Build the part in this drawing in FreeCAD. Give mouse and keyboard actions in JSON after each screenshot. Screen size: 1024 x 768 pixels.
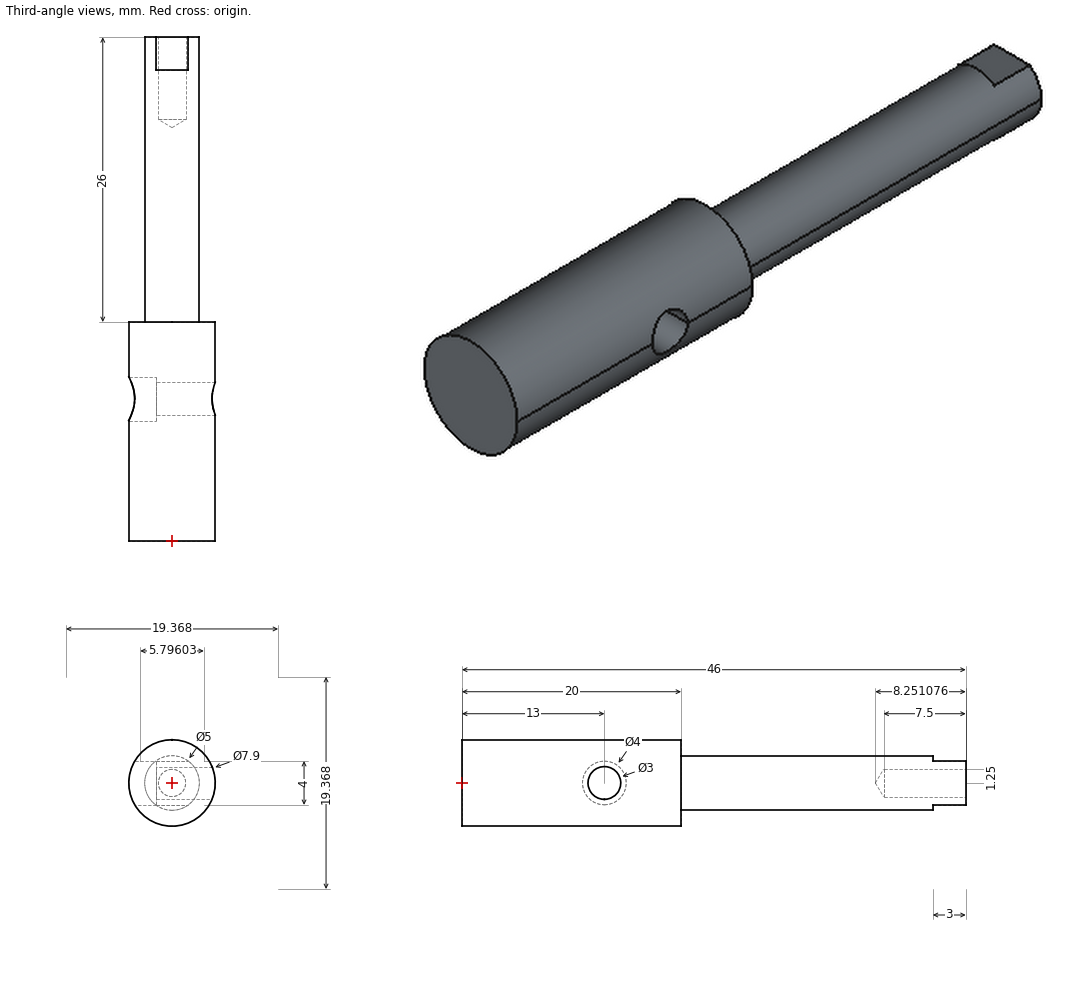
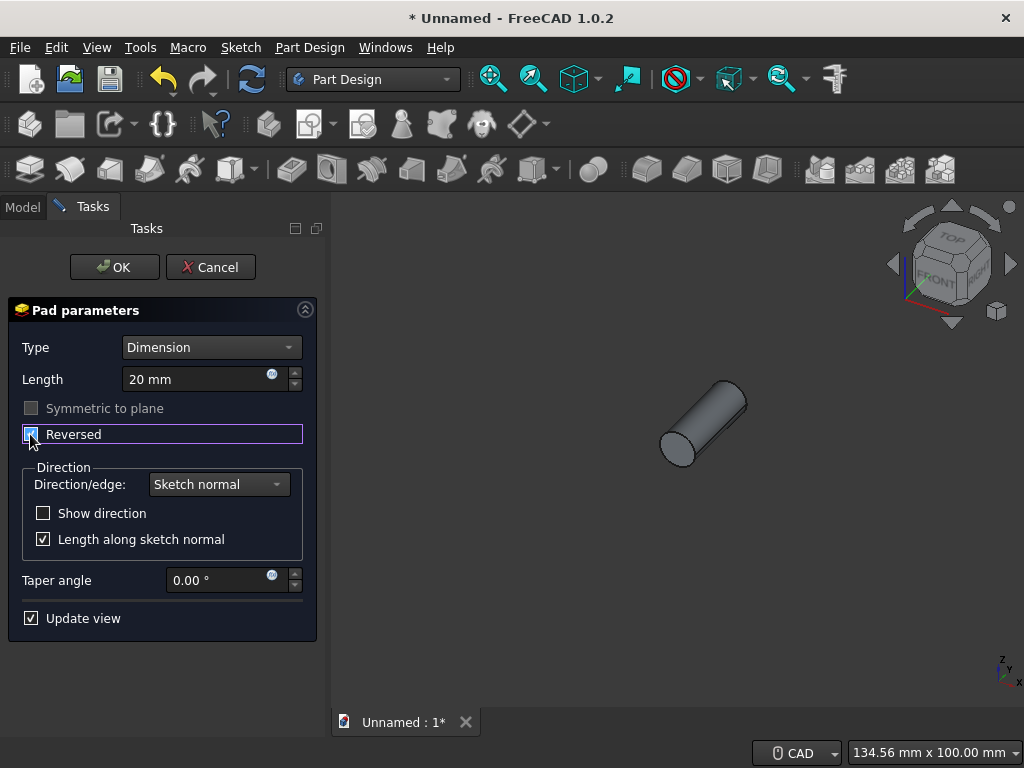
{"action": "left_click", "coordinate": [115, 267]}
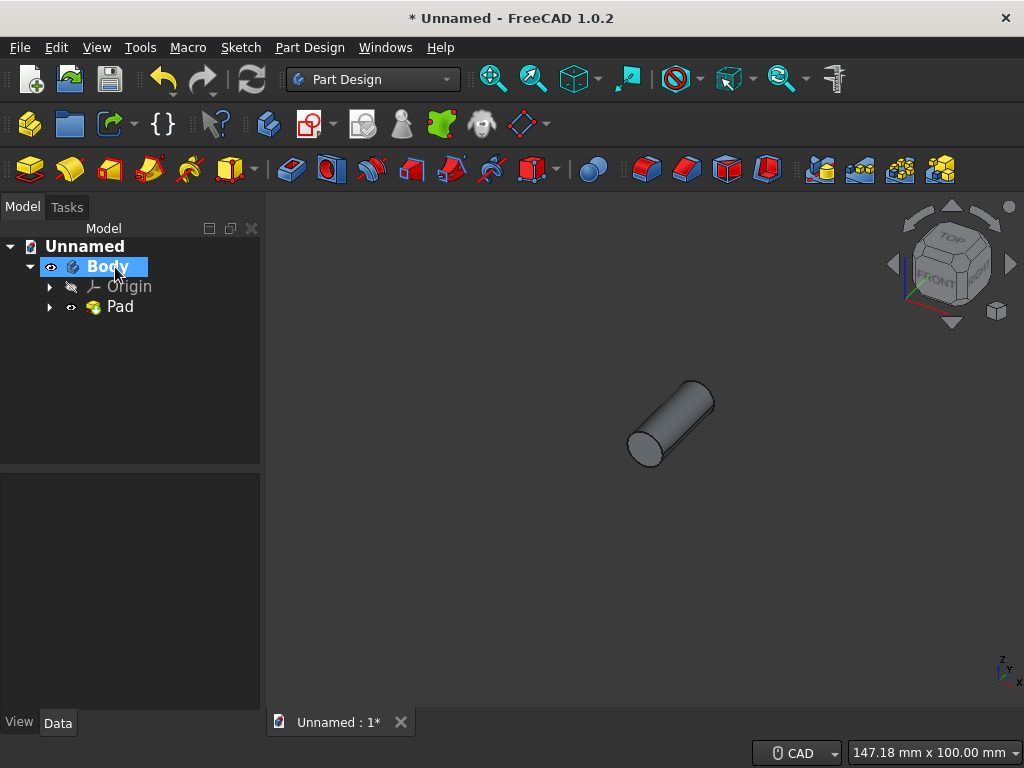
{"action": "left_click", "coordinate": [494, 80]}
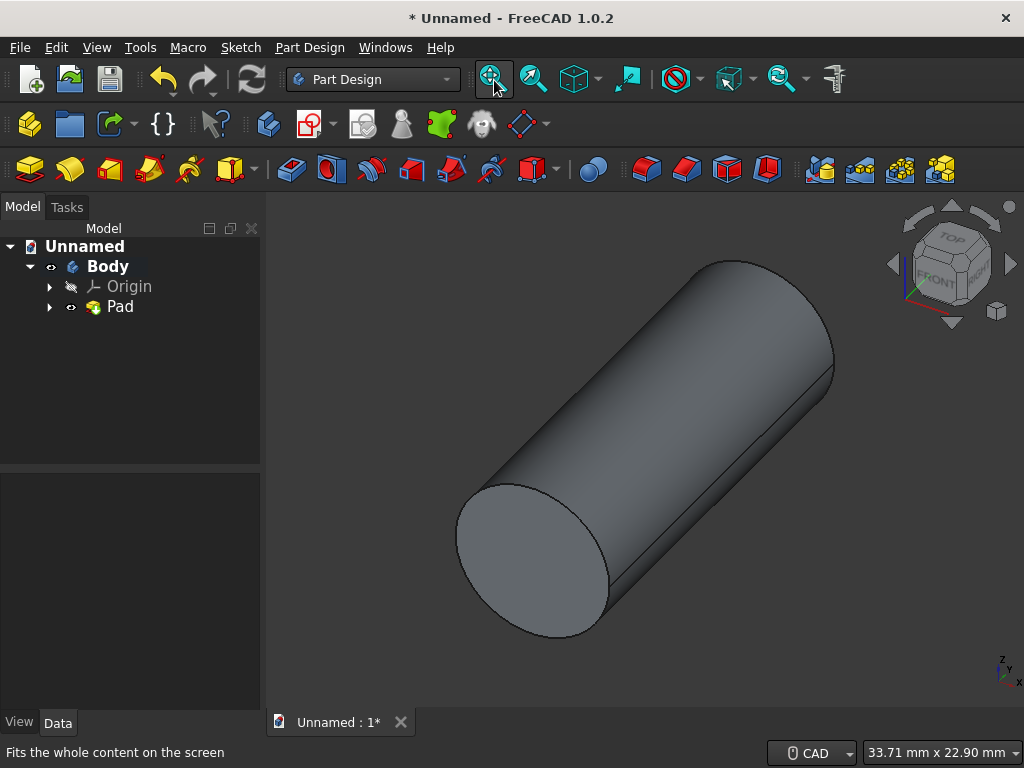
{"action": "key", "text": "4"}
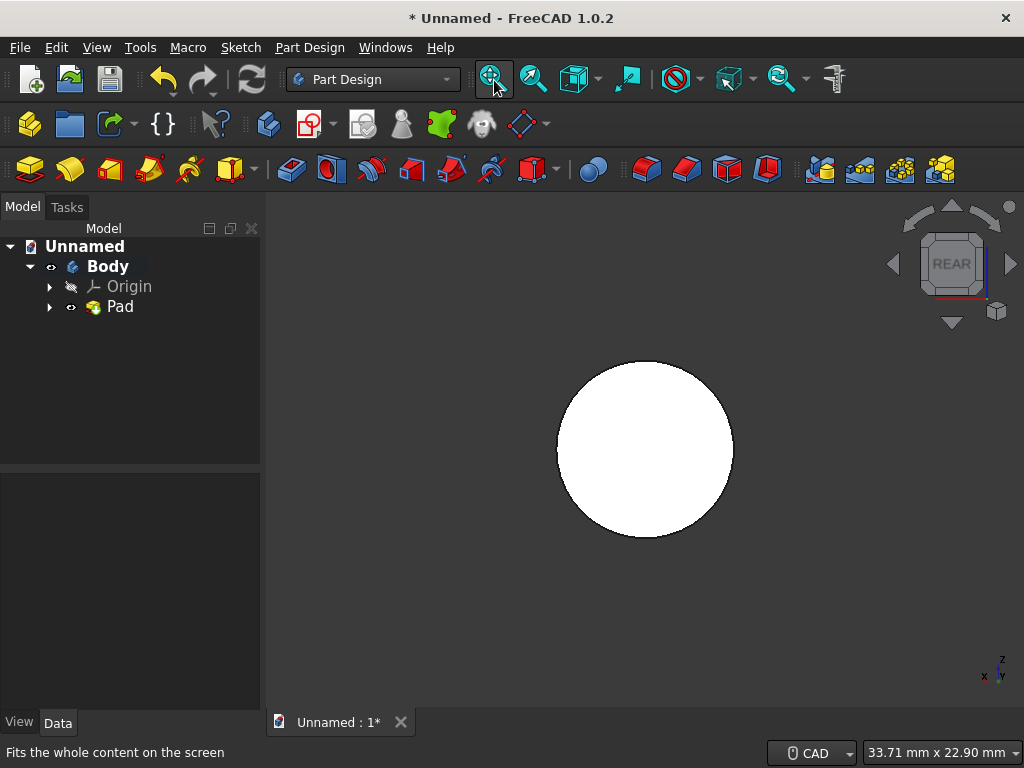
{"action": "left_click", "coordinate": [494, 80]}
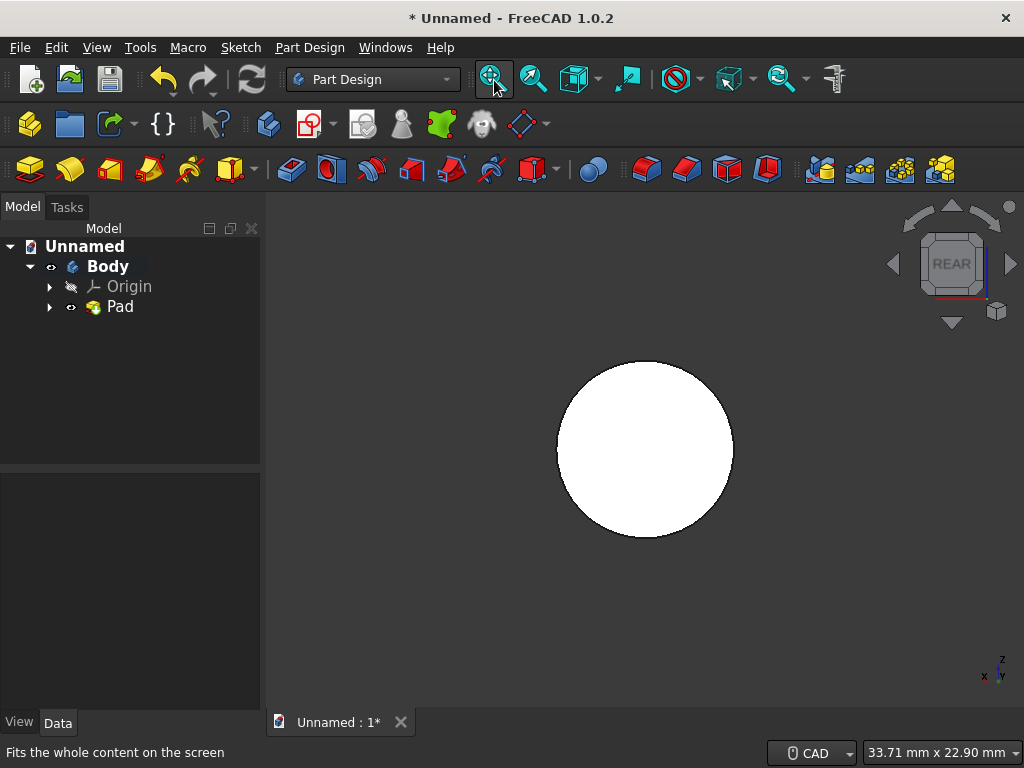
{"action": "left_click", "coordinate": [645, 449]}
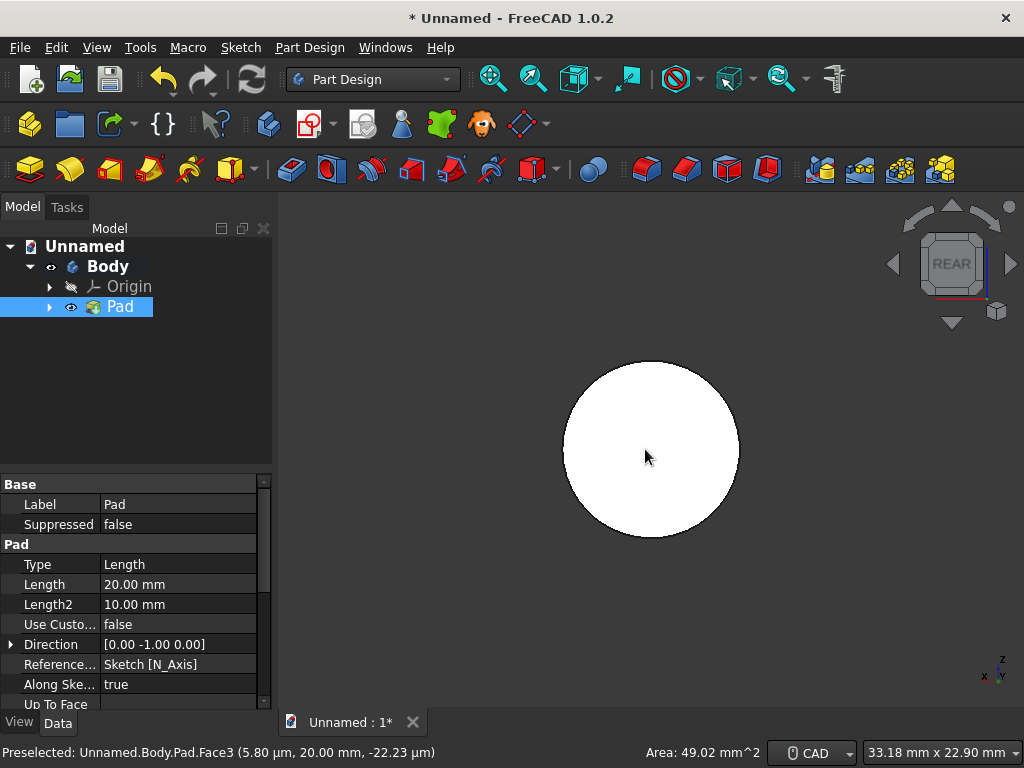
{"action": "left_click", "coordinate": [310, 124]}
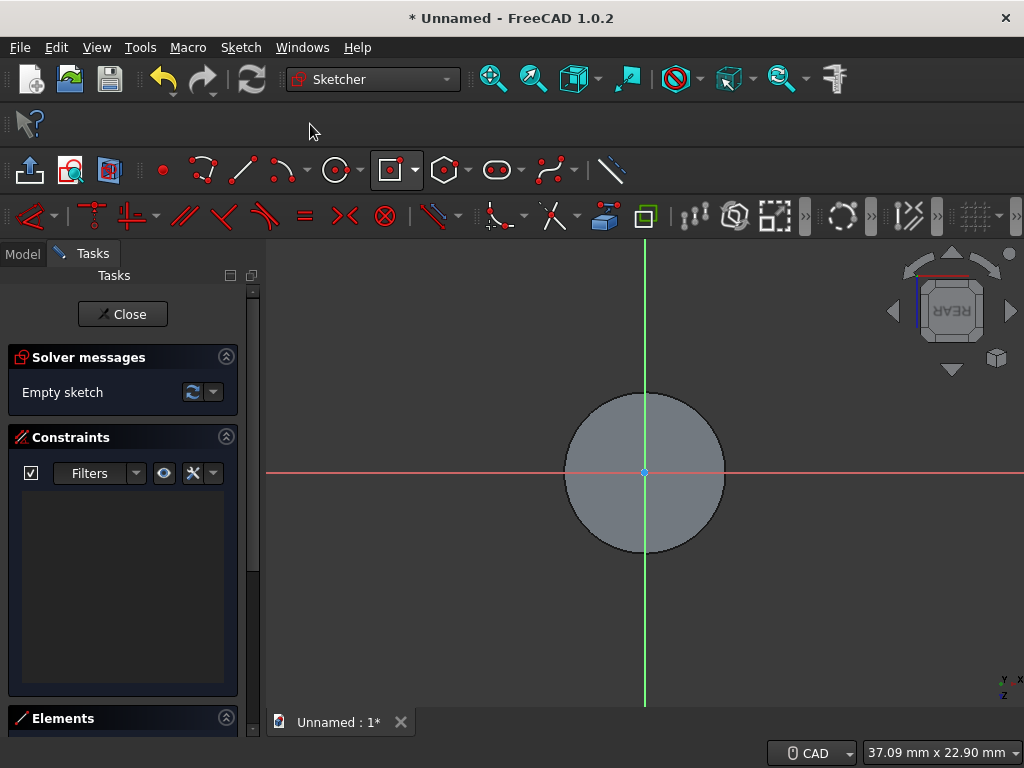
{"action": "scroll", "coordinate": [685, 473], "scroll_direction": "up", "scroll_amount": 5}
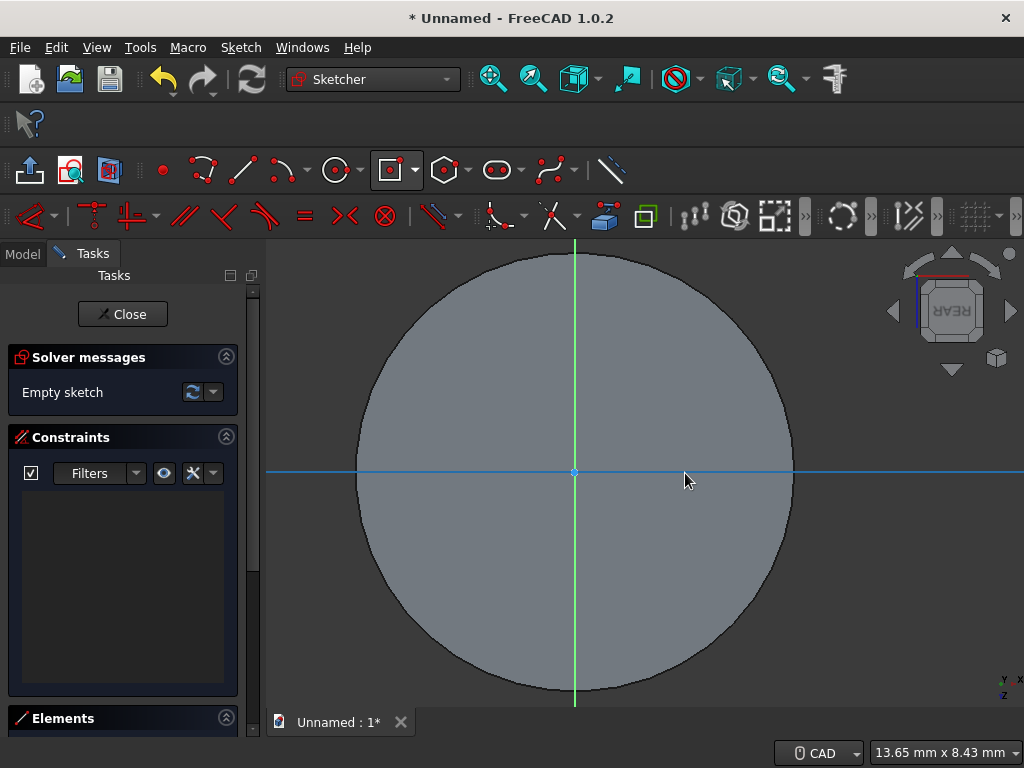
{"action": "left_click", "coordinate": [336, 170]}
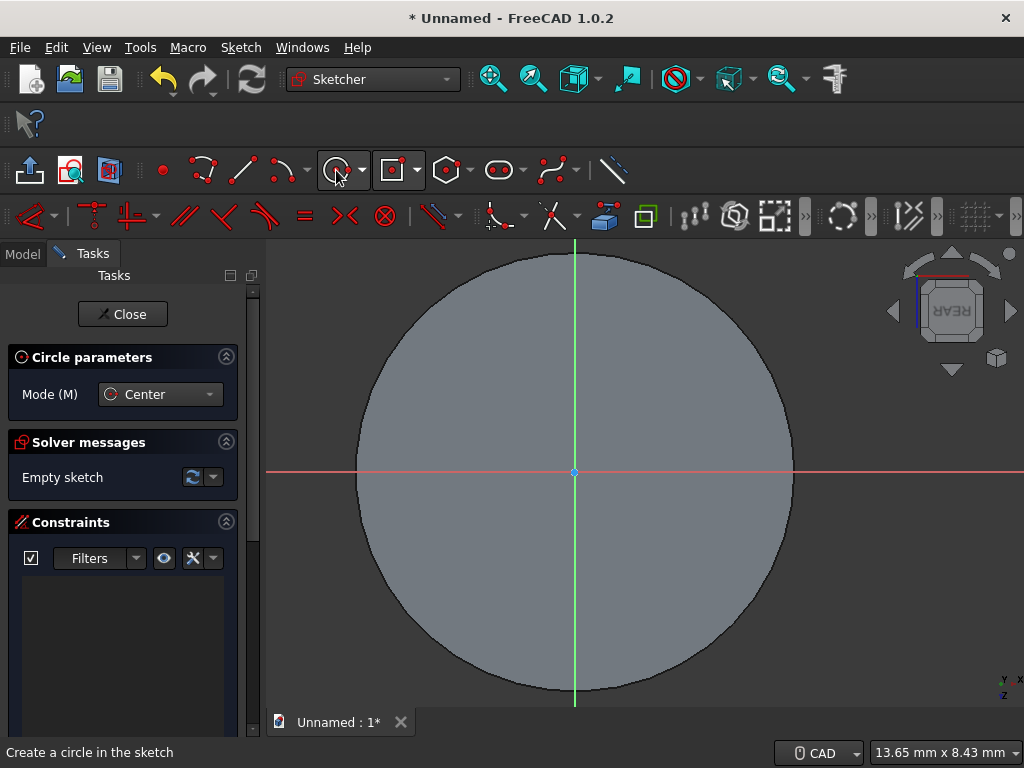
{"action": "left_click", "coordinate": [575, 472]}
{"action": "mouse_move", "coordinate": [673, 374]}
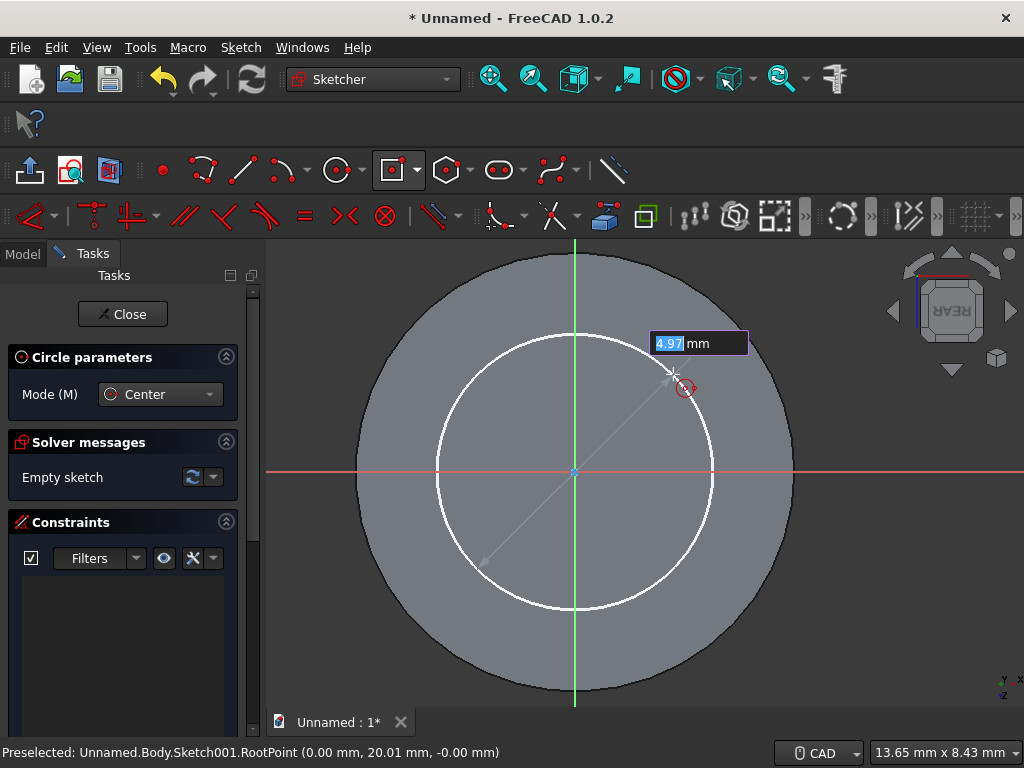
{"action": "type", "text": "5"}
{"action": "key", "text": "Return"}
{"action": "key", "text": "Escape"}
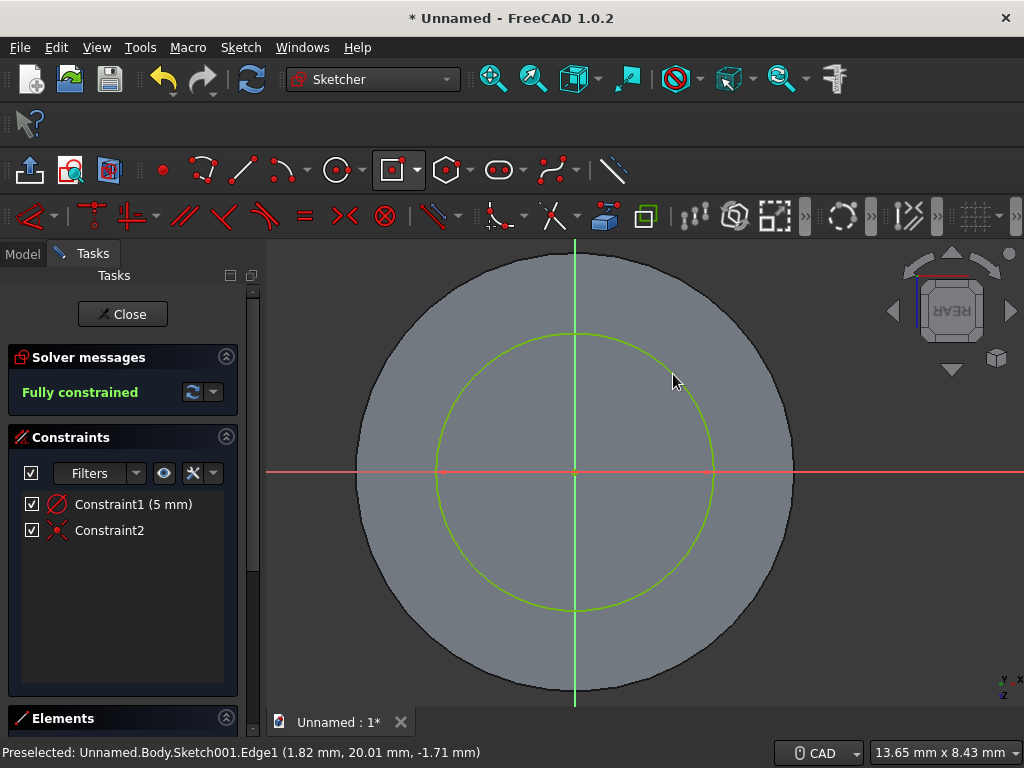
{"action": "left_click", "coordinate": [123, 314]}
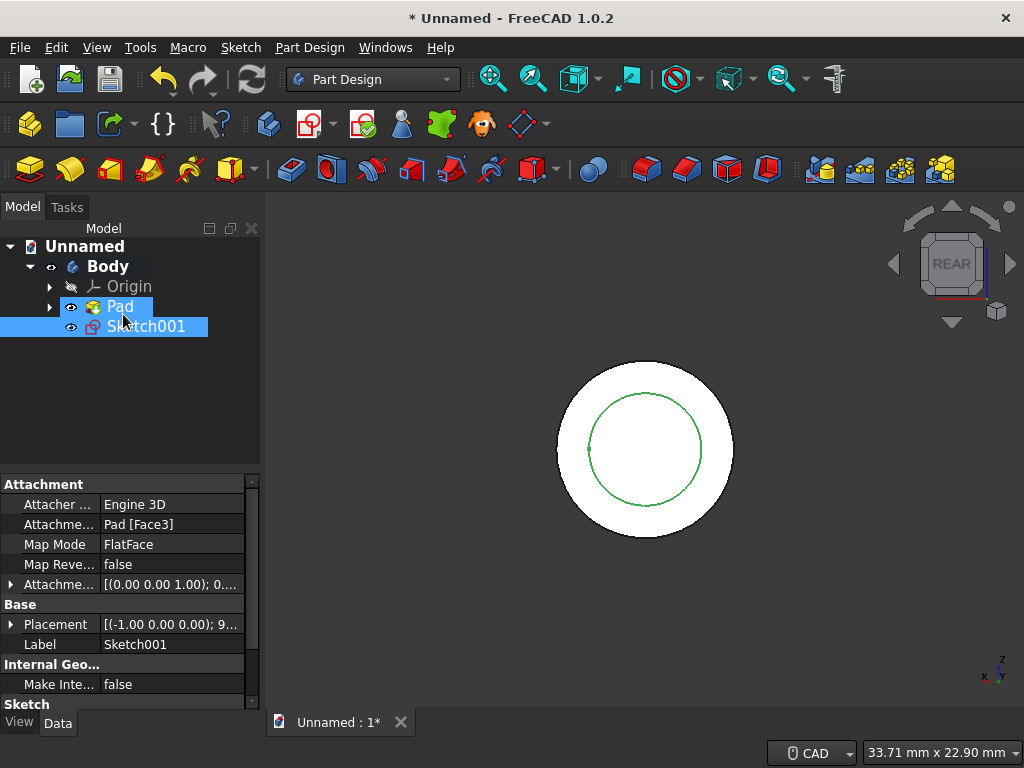
{"action": "left_click", "coordinate": [30, 170]}